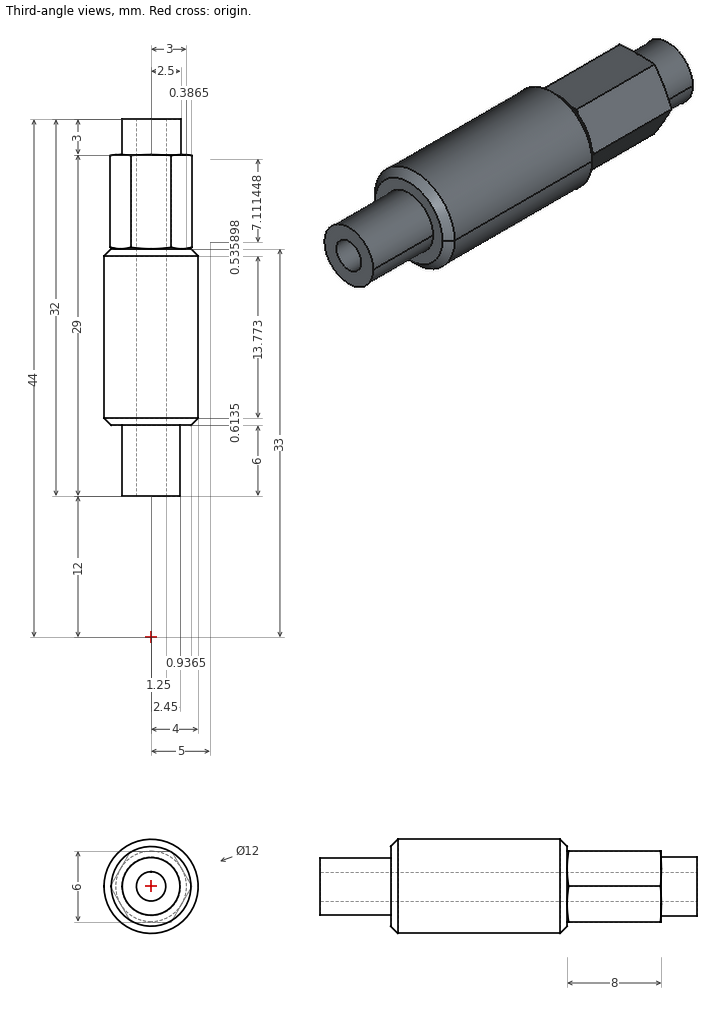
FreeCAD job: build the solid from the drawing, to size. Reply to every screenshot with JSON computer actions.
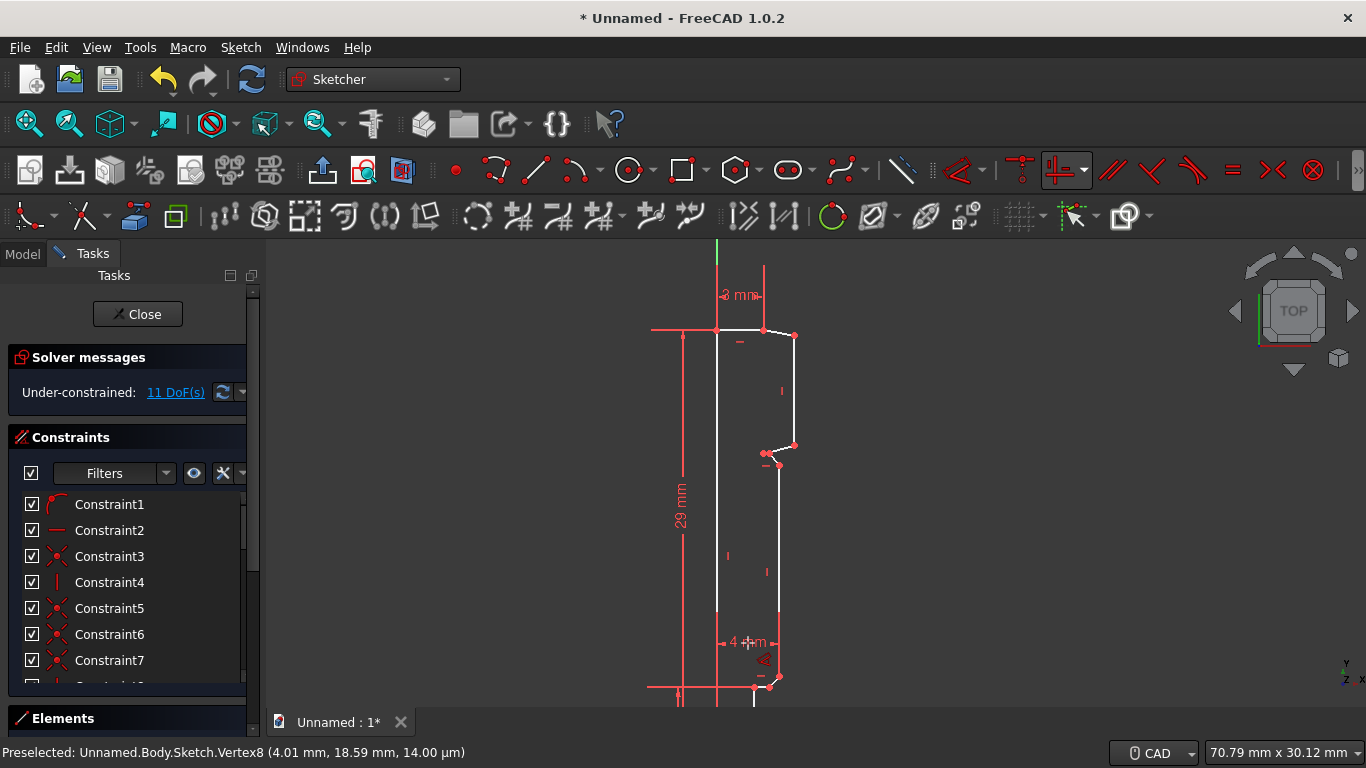
{"action": "scroll", "coordinate": [763, 454], "scroll_direction": "up", "scroll_amount": 4}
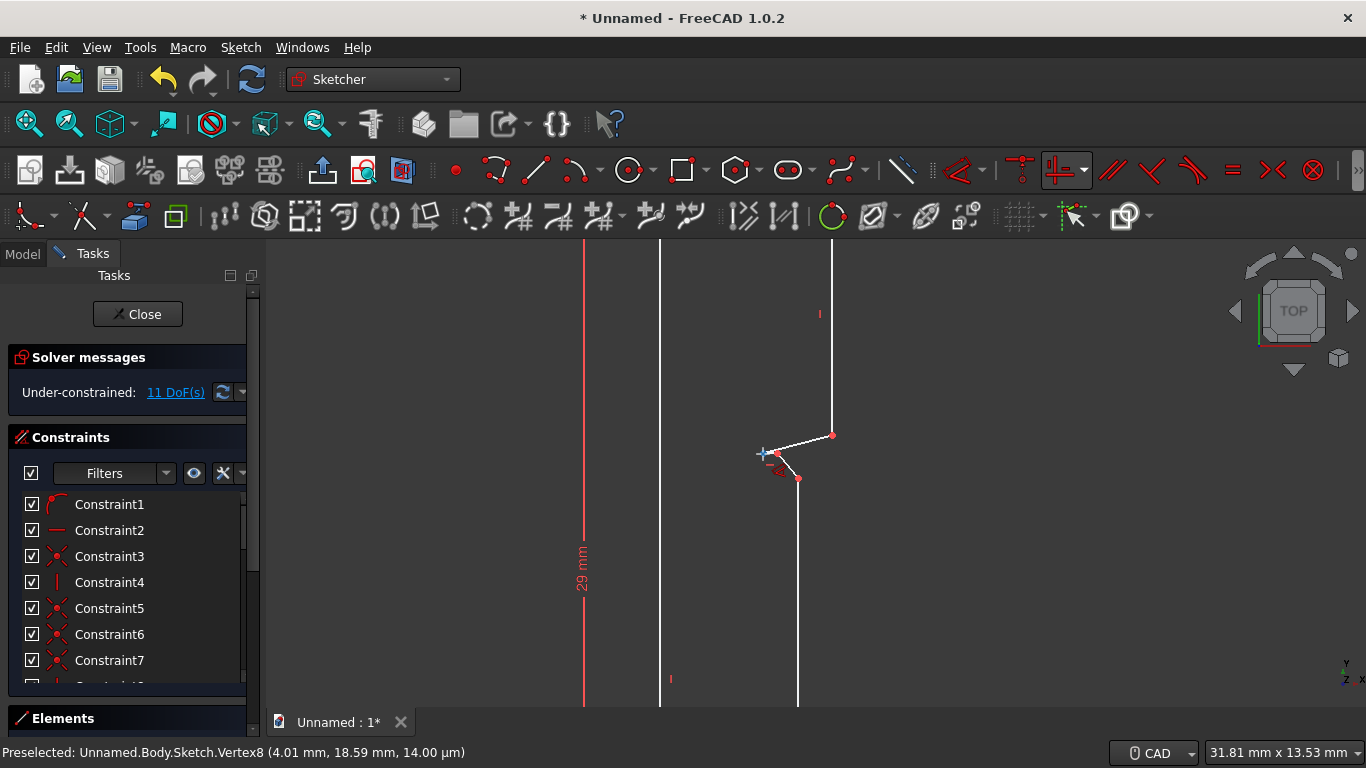
{"action": "left_click", "coordinate": [764, 453]}
{"action": "left_click", "coordinate": [712, 419]}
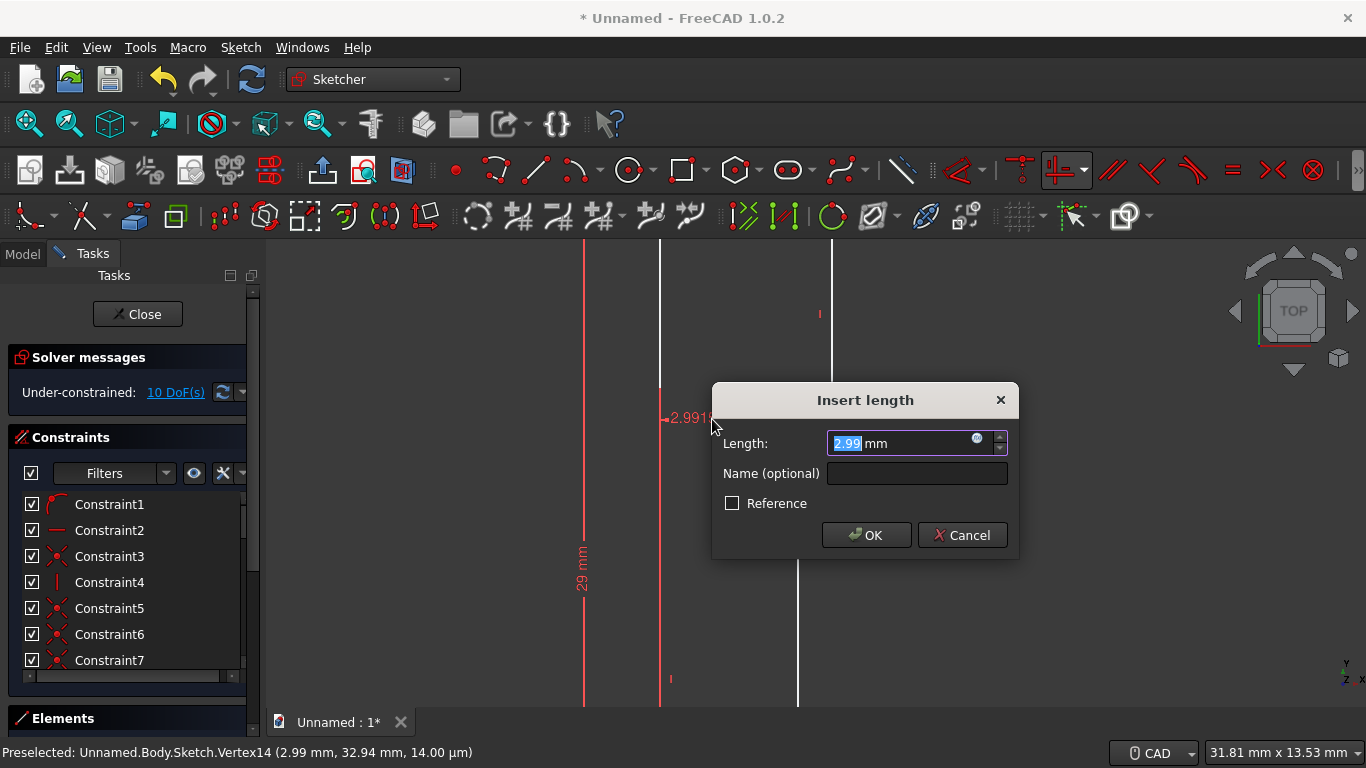
{"action": "type", "text": "3"}
{"action": "key", "text": "Return"}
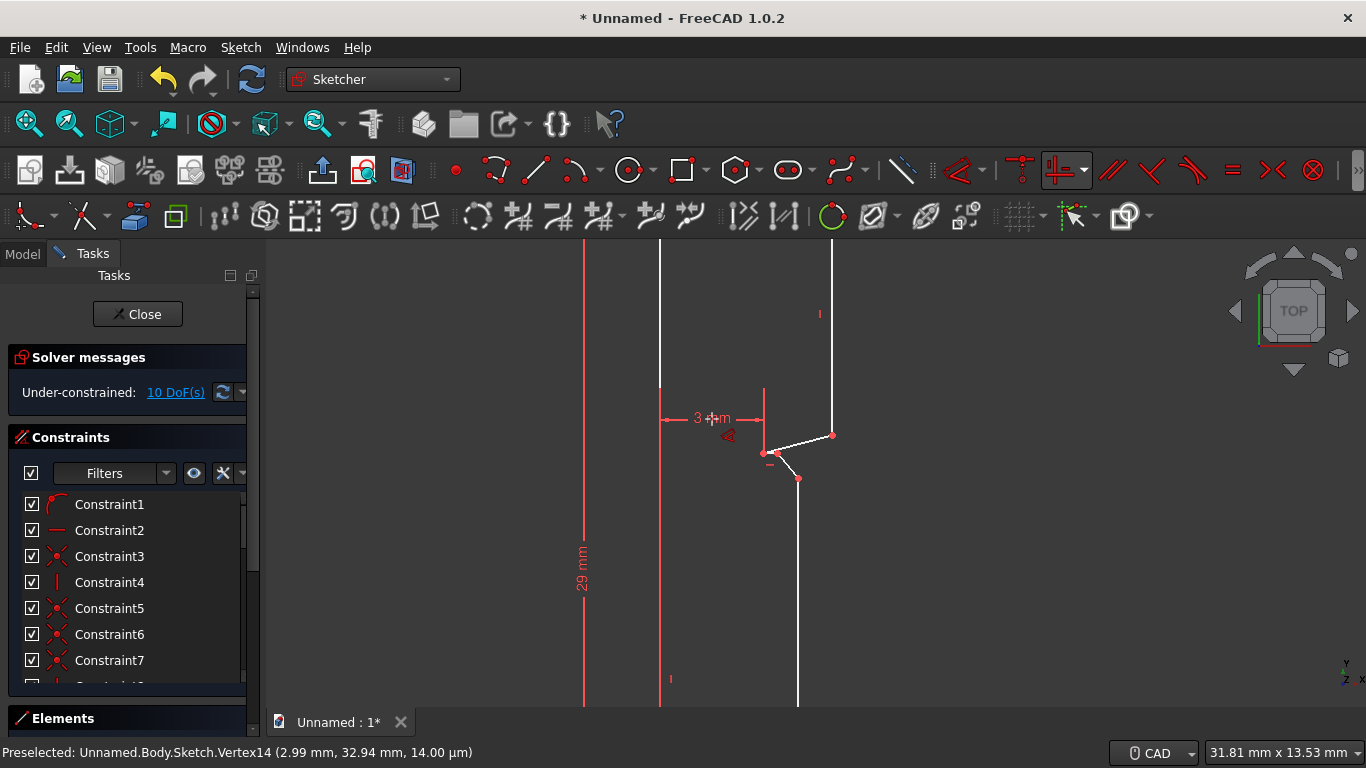
{"action": "scroll", "coordinate": [748, 369], "scroll_direction": "down", "scroll_amount": 8}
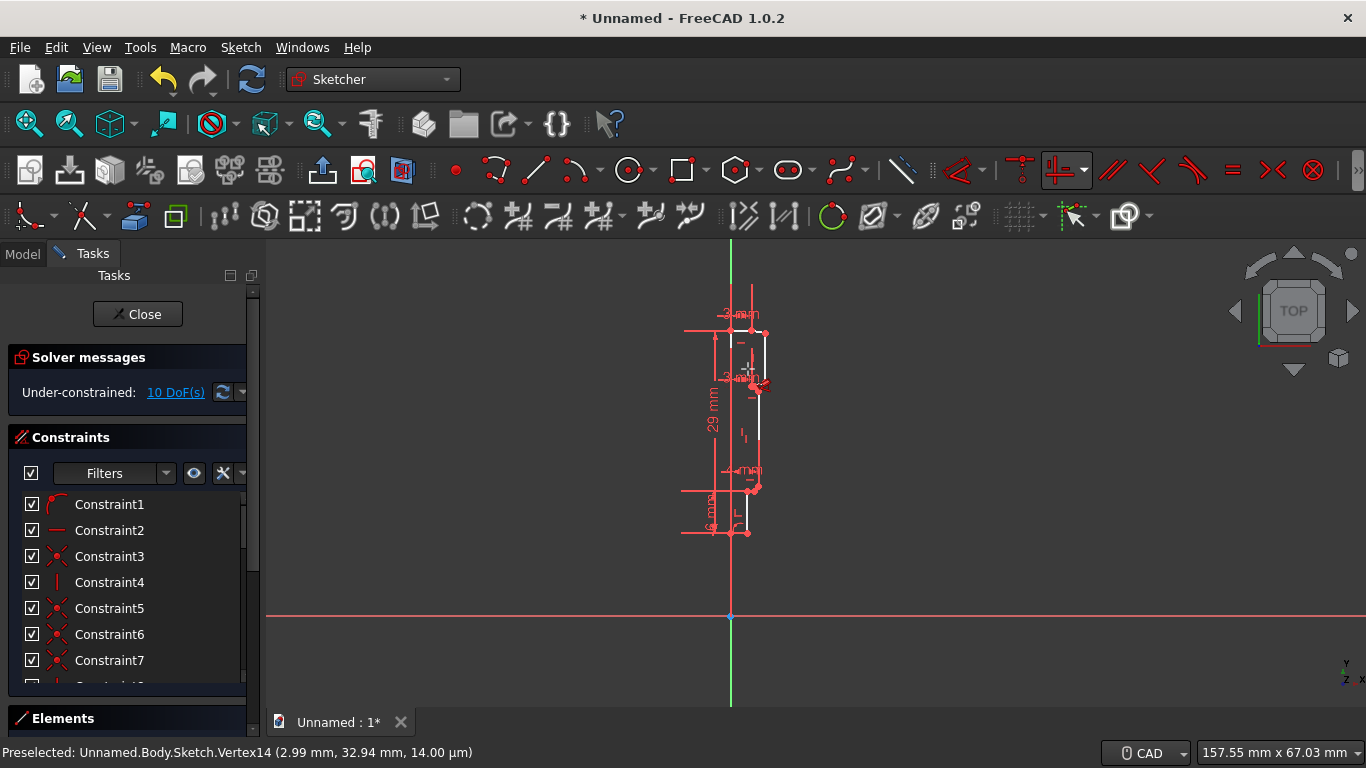
{"action": "left_click", "coordinate": [765, 383]}
{"action": "left_click", "coordinate": [748, 650]}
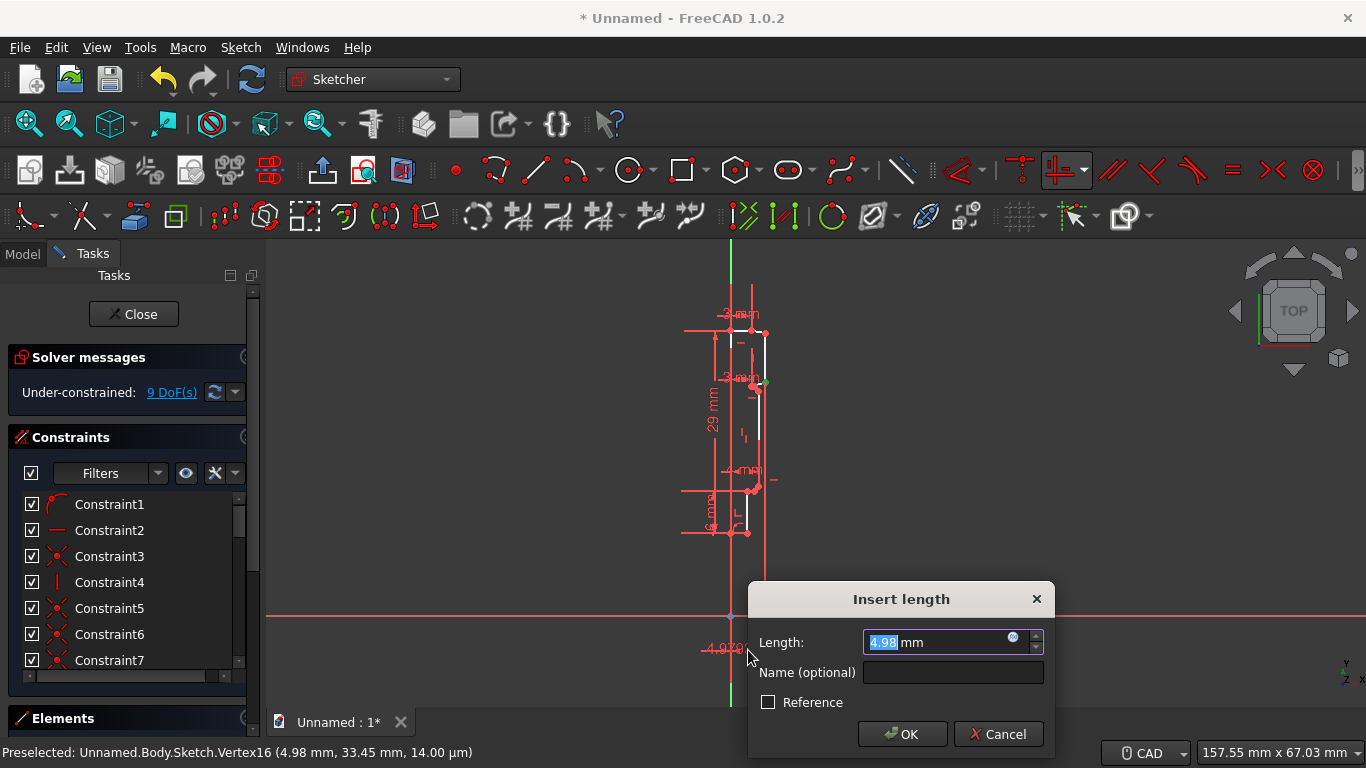
{"action": "type", "text": "5"}
{"action": "key", "text": "Return"}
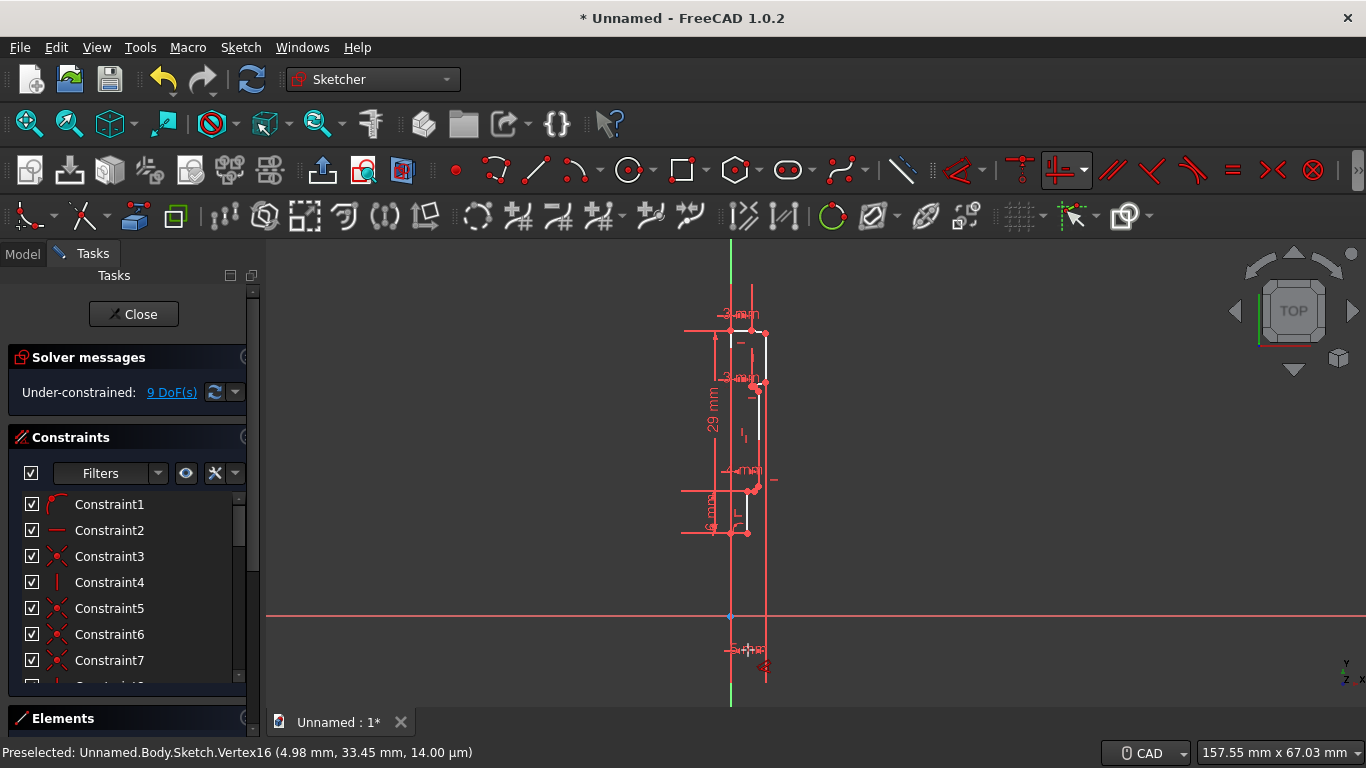
{"action": "left_click", "coordinate": [731, 533]}
{"action": "left_click", "coordinate": [697, 575]}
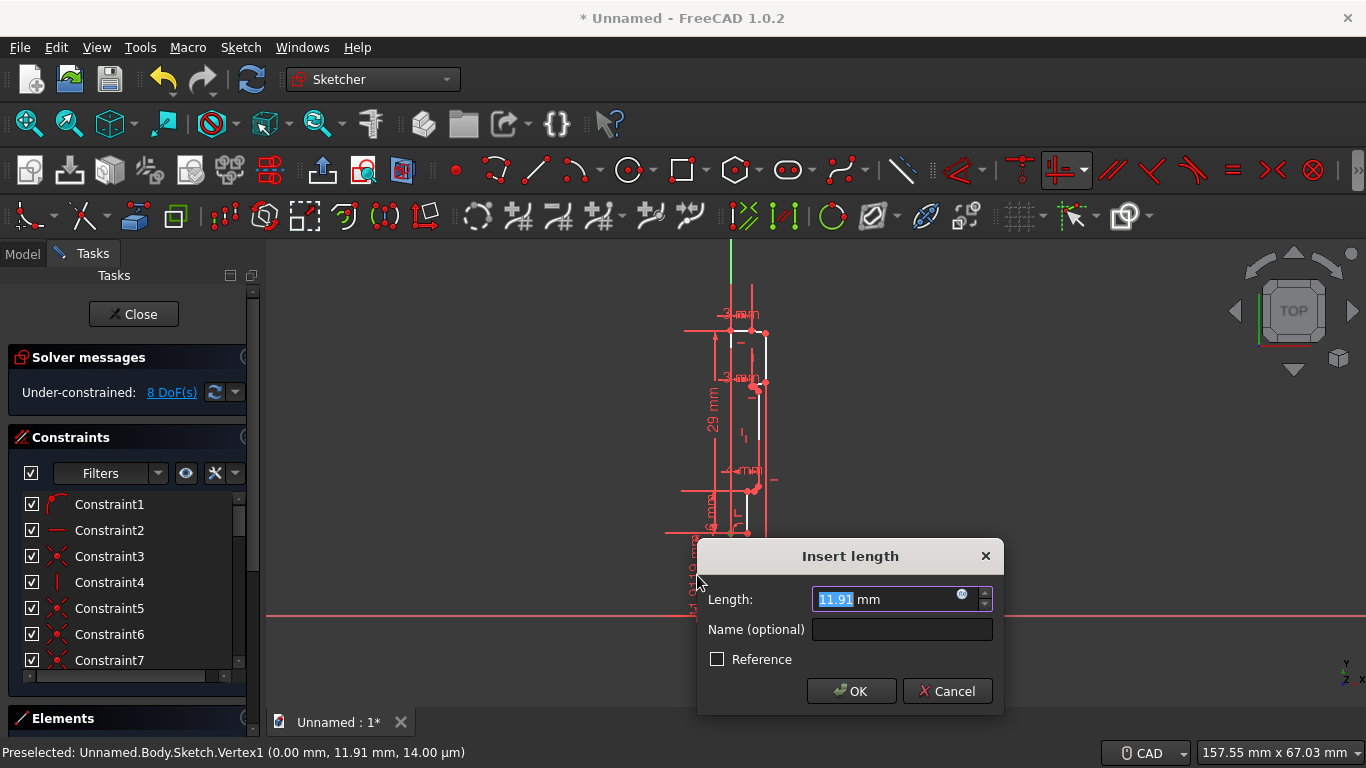
{"action": "type", "text": "12"}
{"action": "key", "text": "Return"}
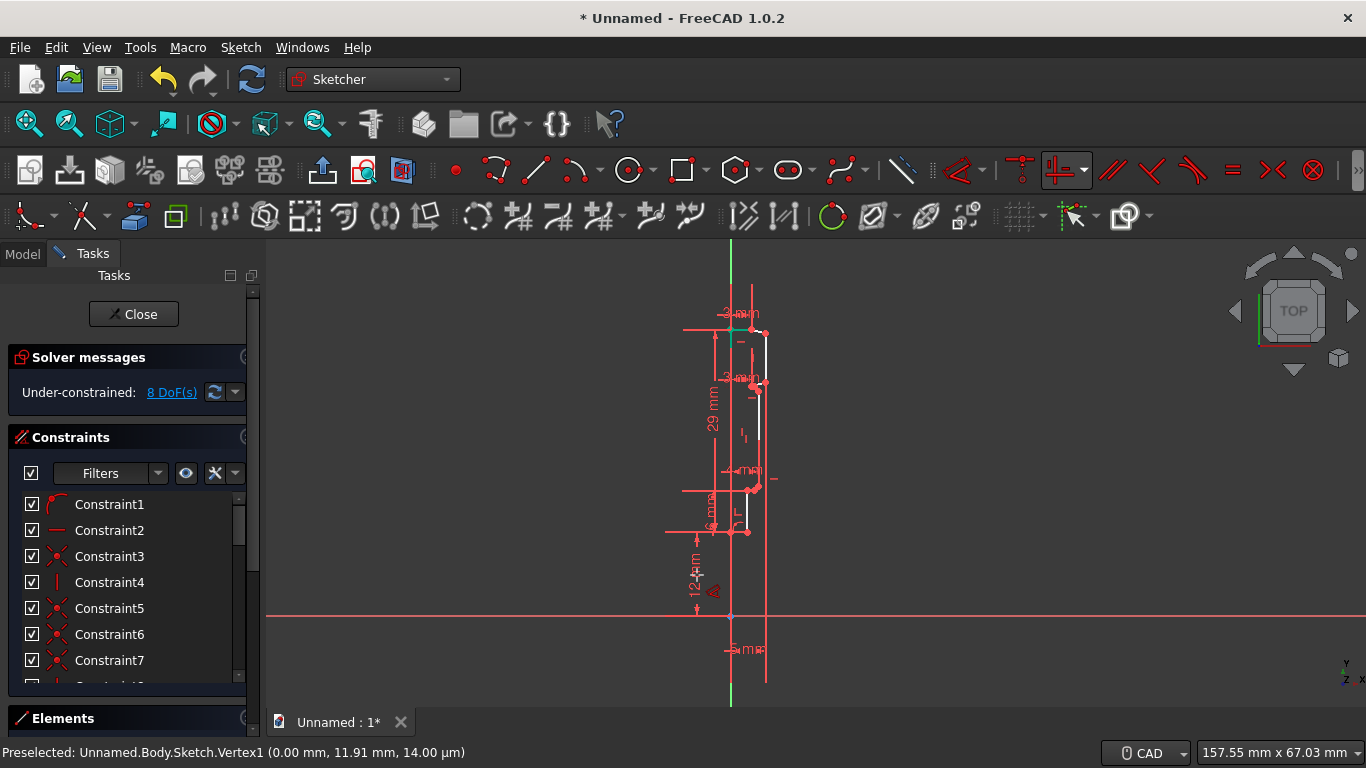
{"action": "scroll", "coordinate": [754, 386], "scroll_direction": "up", "scroll_amount": 8}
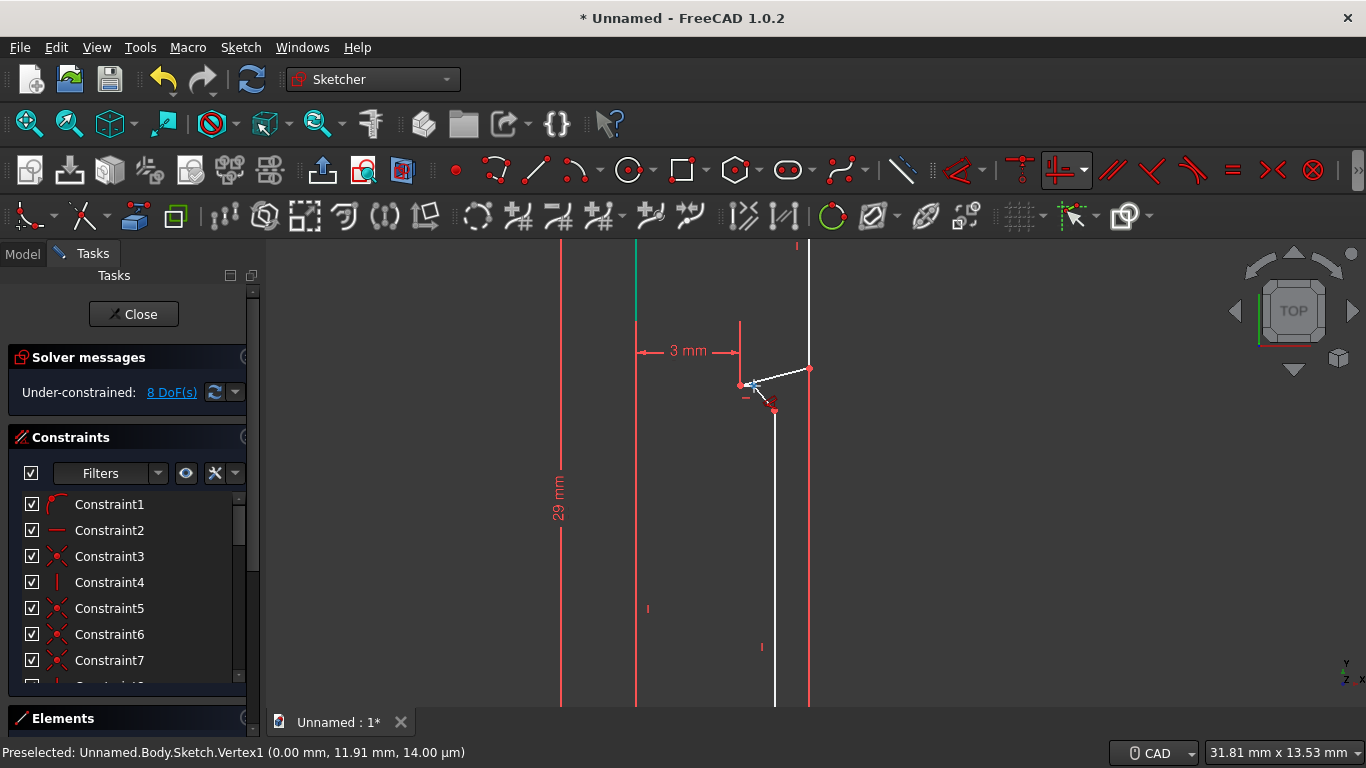
{"action": "left_click", "coordinate": [754, 386]}
{"action": "left_click", "coordinate": [602, 532]}